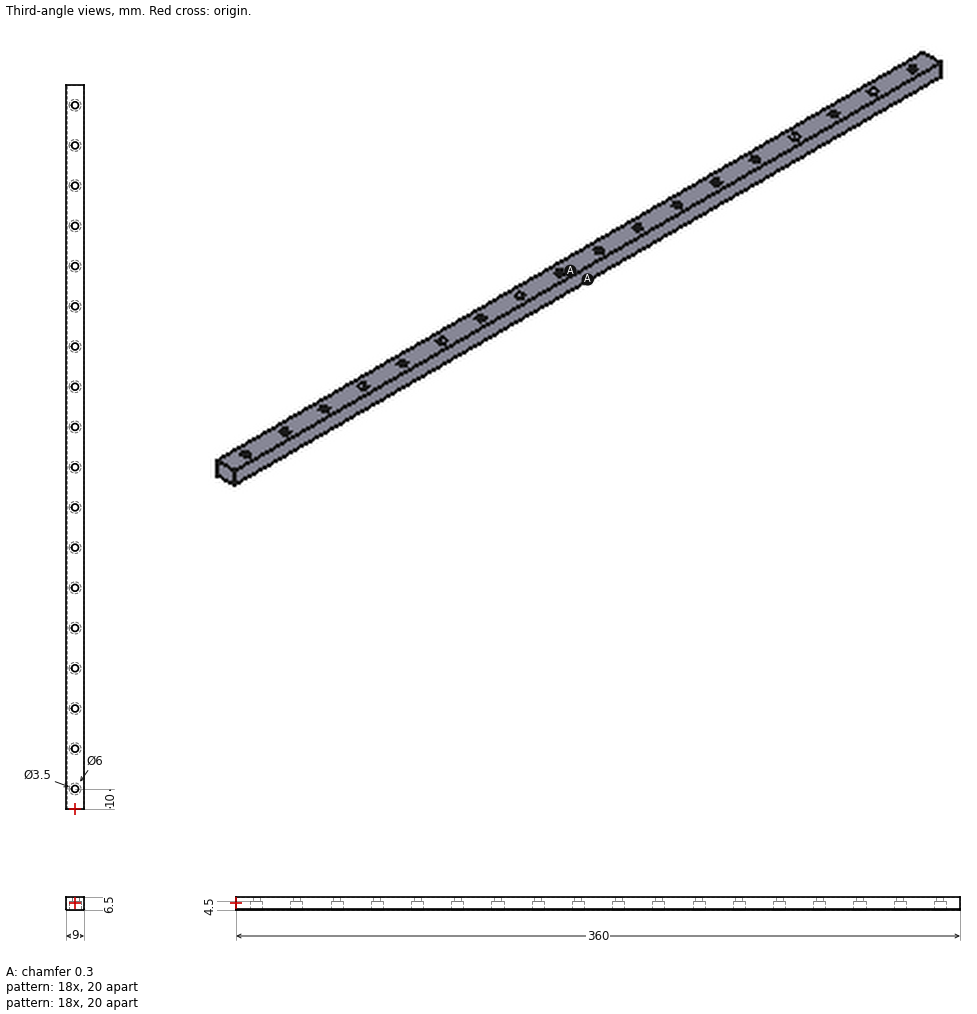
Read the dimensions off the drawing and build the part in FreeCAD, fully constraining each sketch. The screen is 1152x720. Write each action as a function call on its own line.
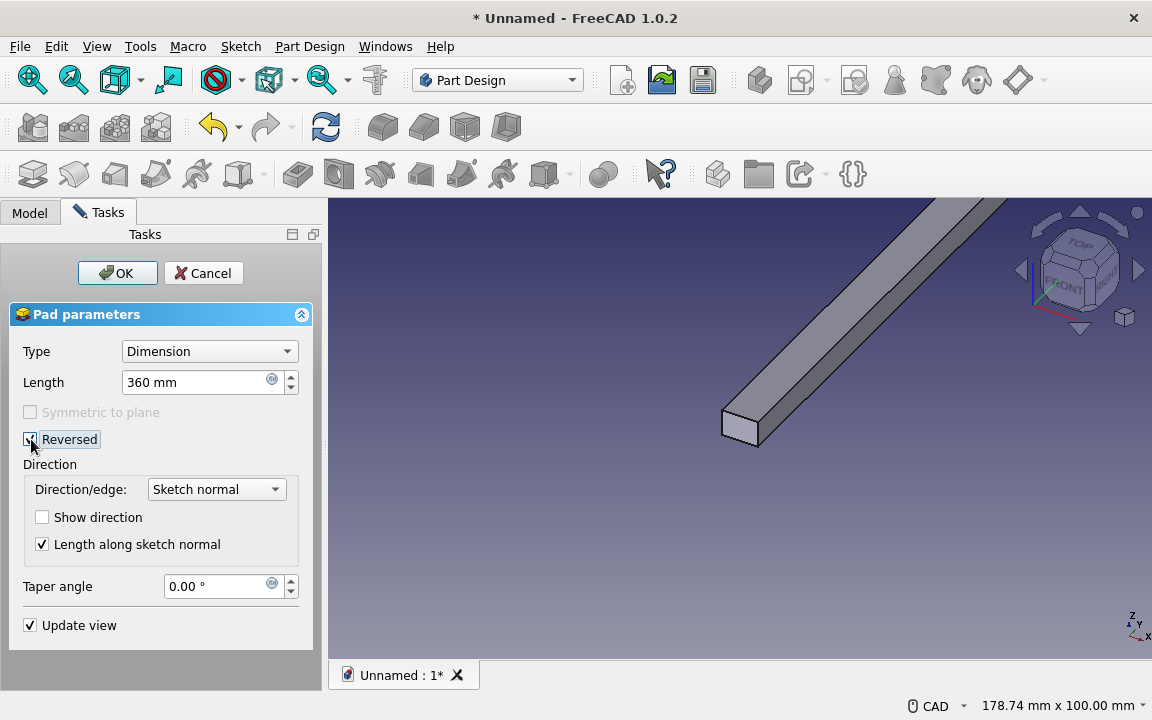
click(118, 273)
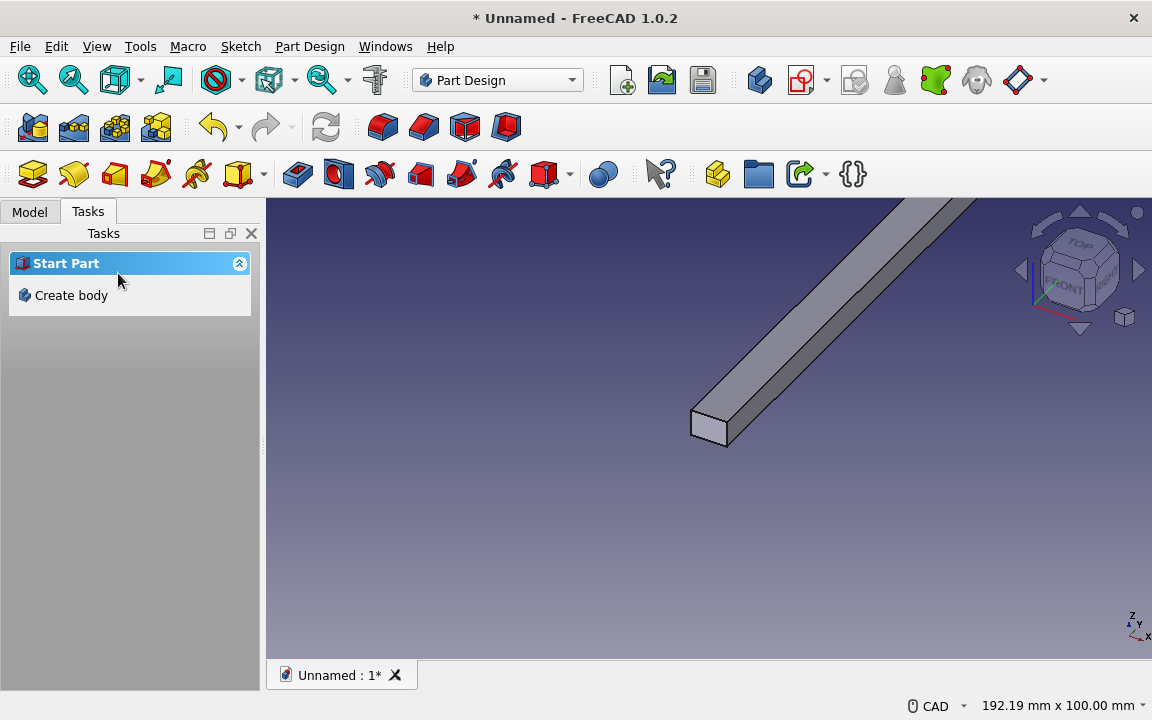
click(33, 80)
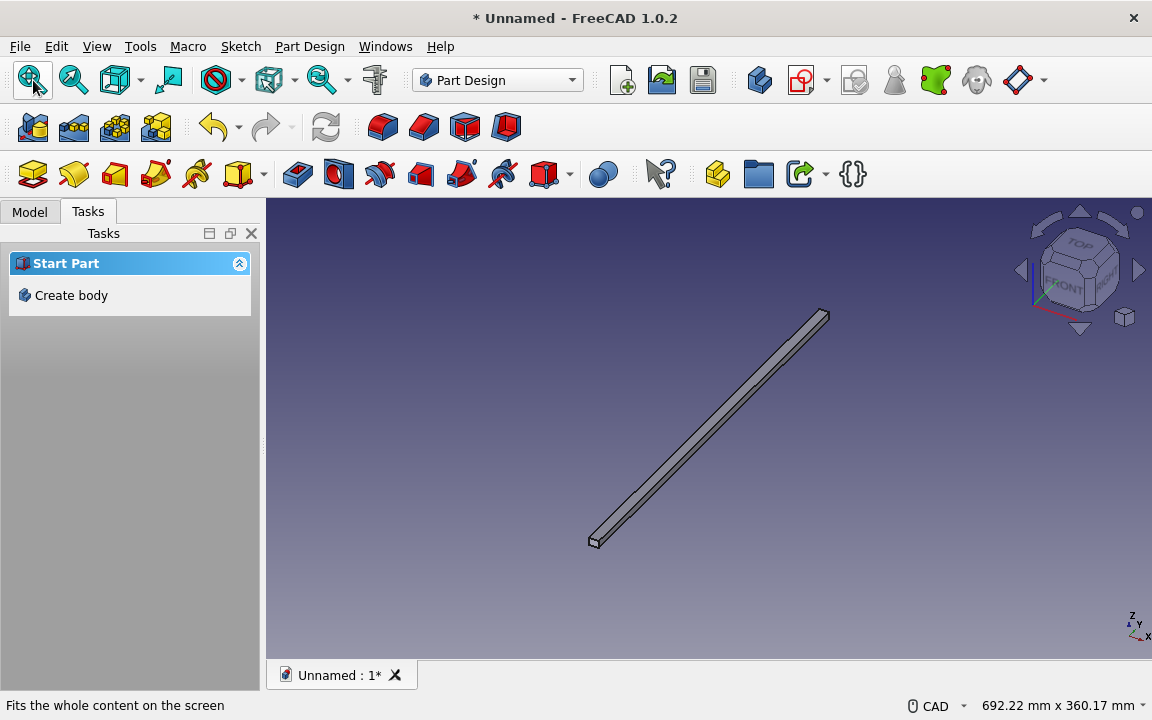
key(0)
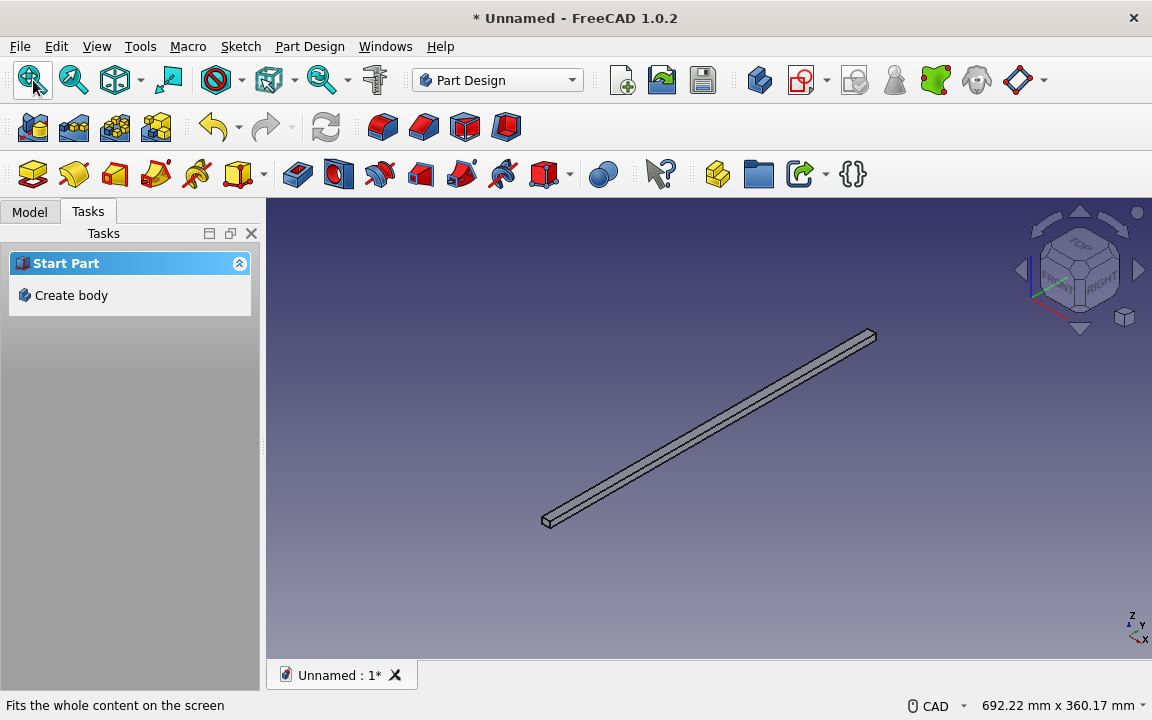
key(v)
key(f)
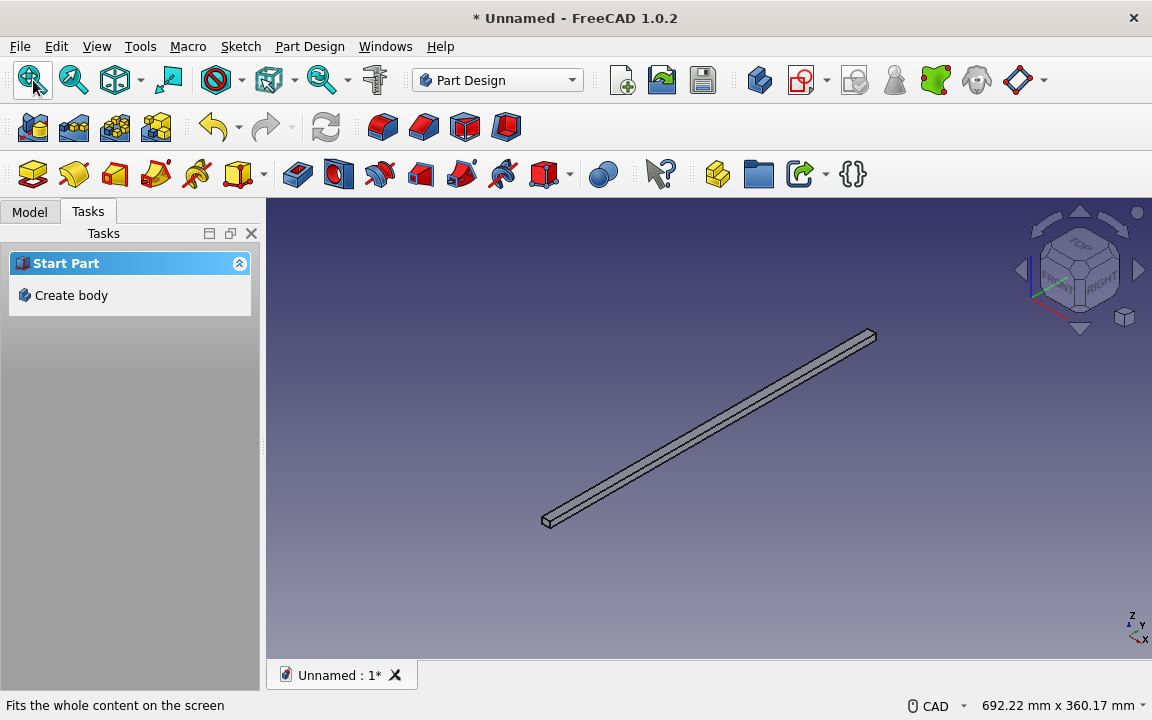
key(2)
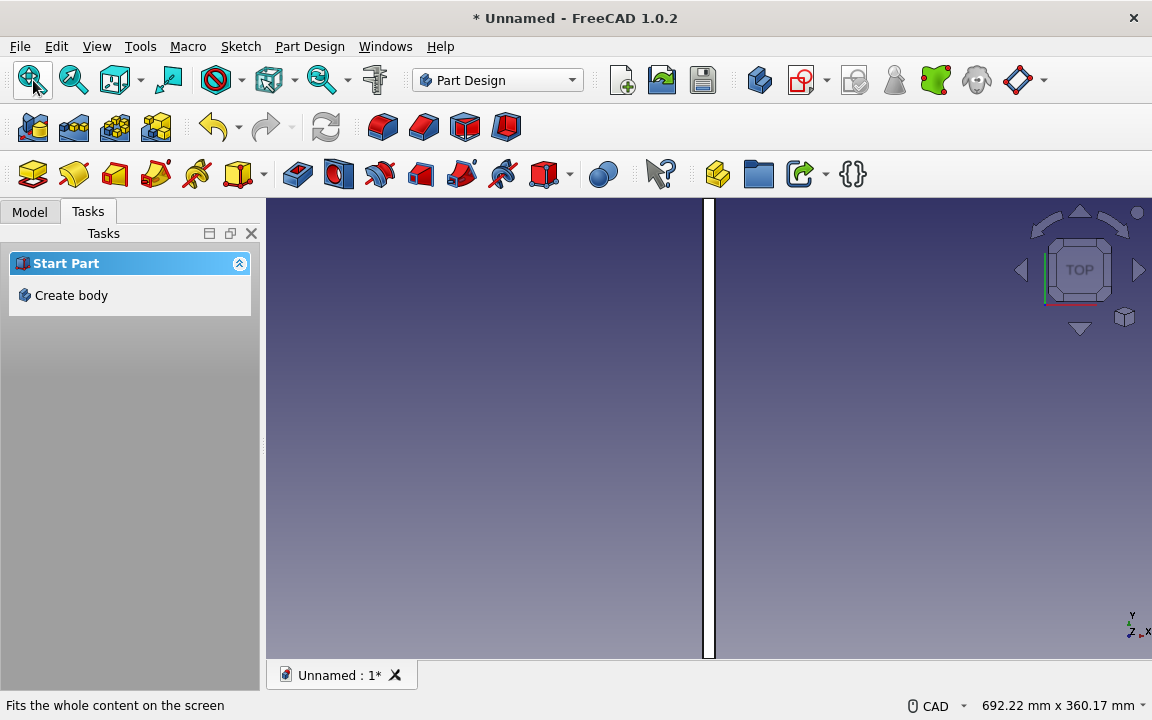
key(v)
key(f)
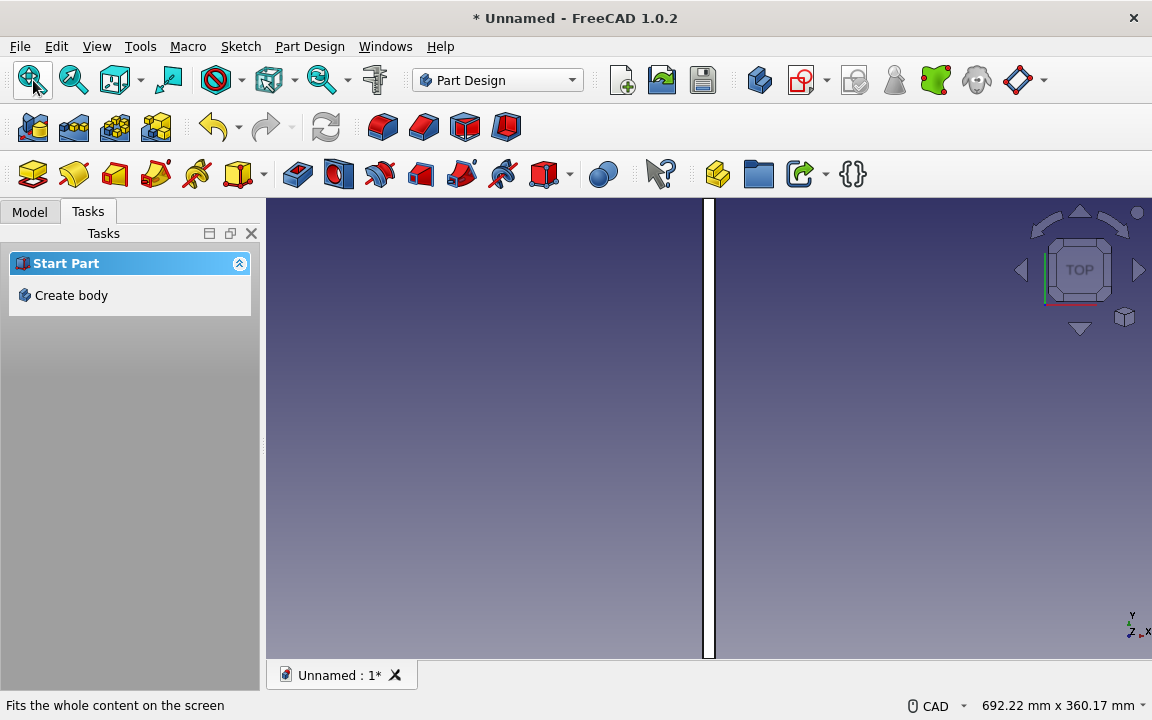
key(1)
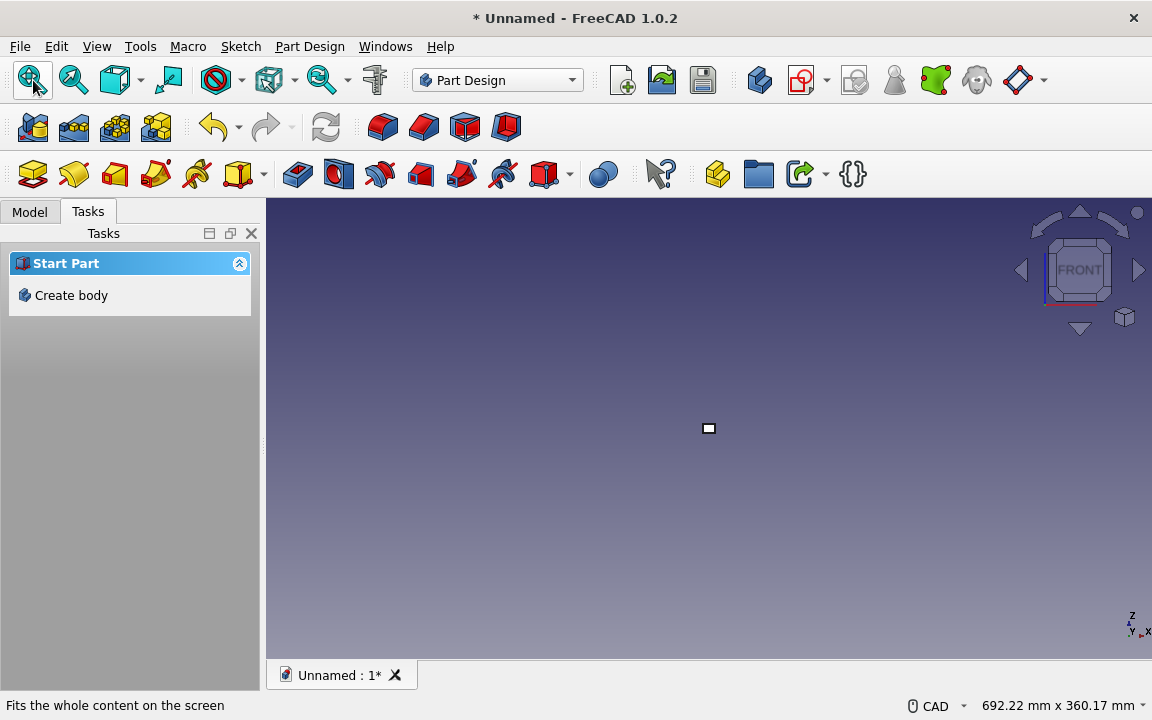
key(v)
key(f)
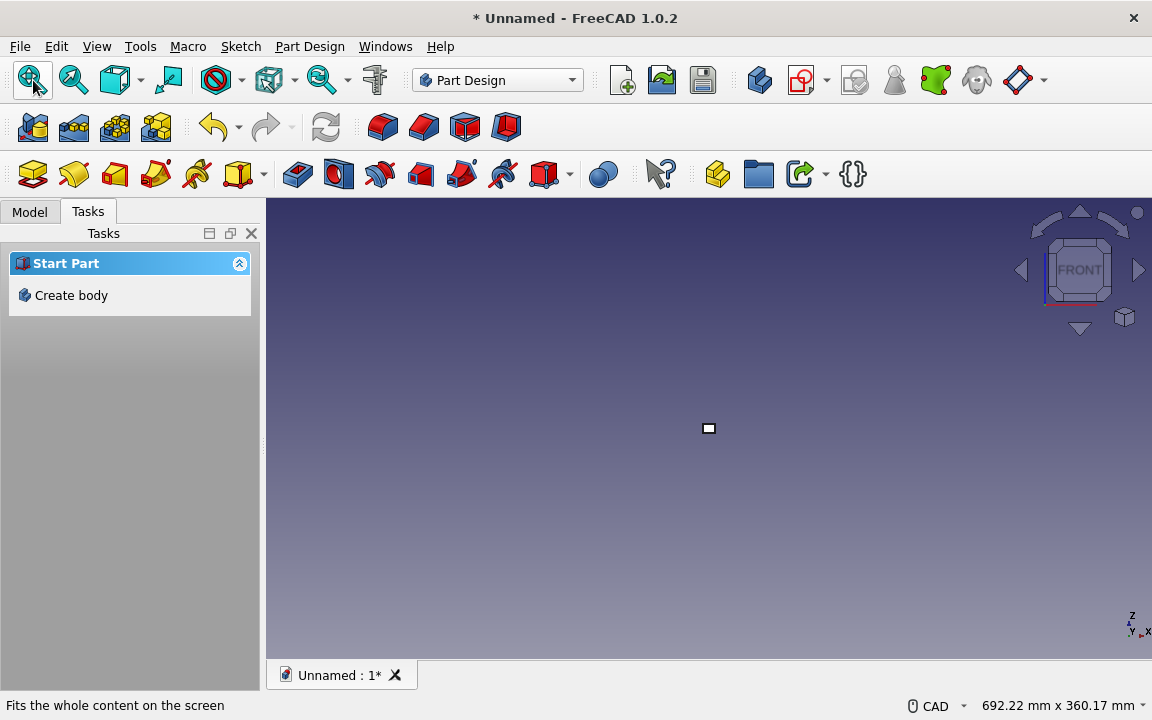
key(3)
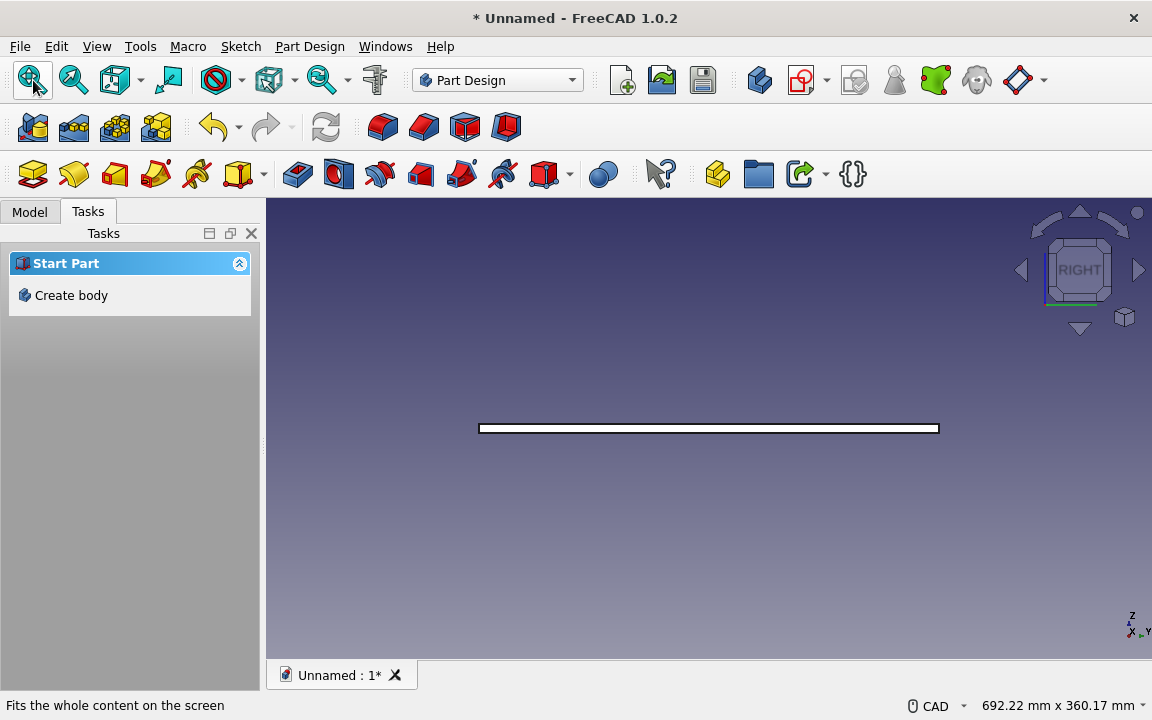
click(709, 432)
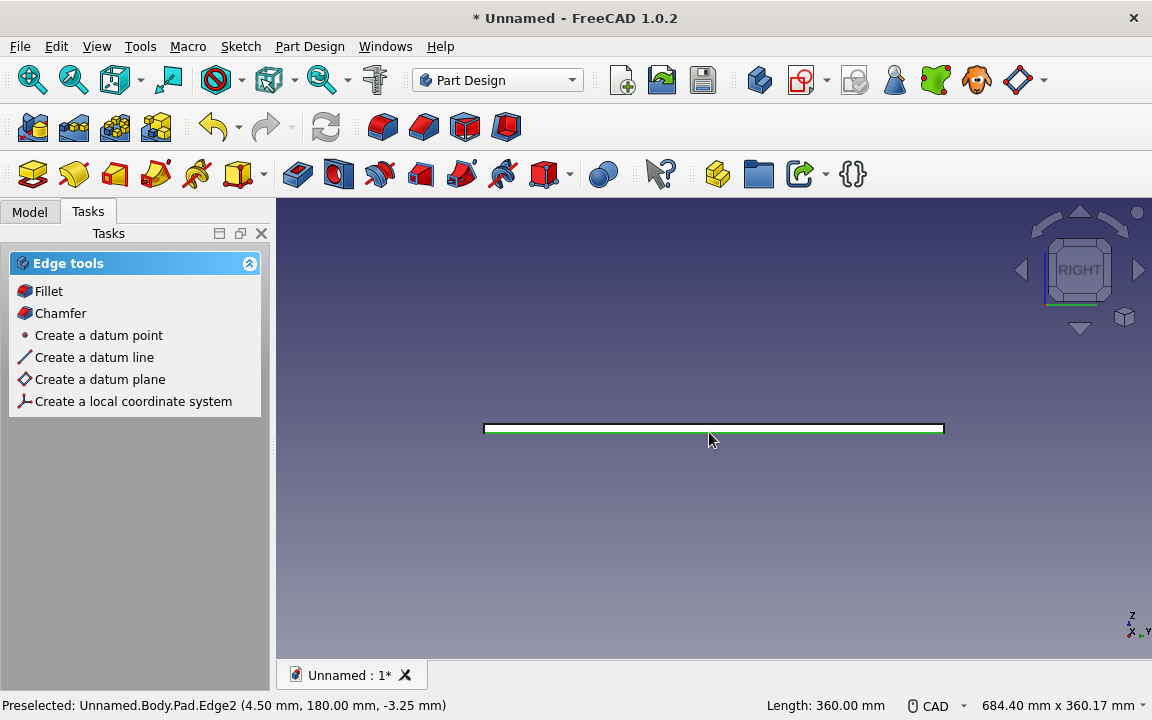
key(5)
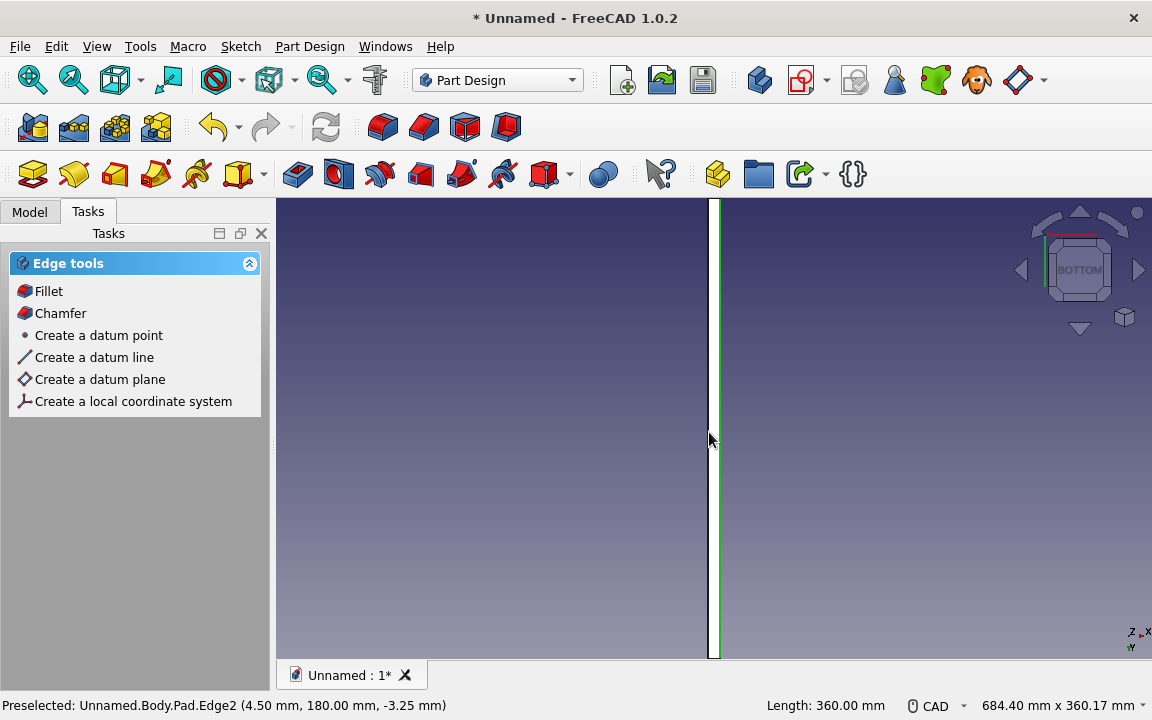
key(v)
key(f)